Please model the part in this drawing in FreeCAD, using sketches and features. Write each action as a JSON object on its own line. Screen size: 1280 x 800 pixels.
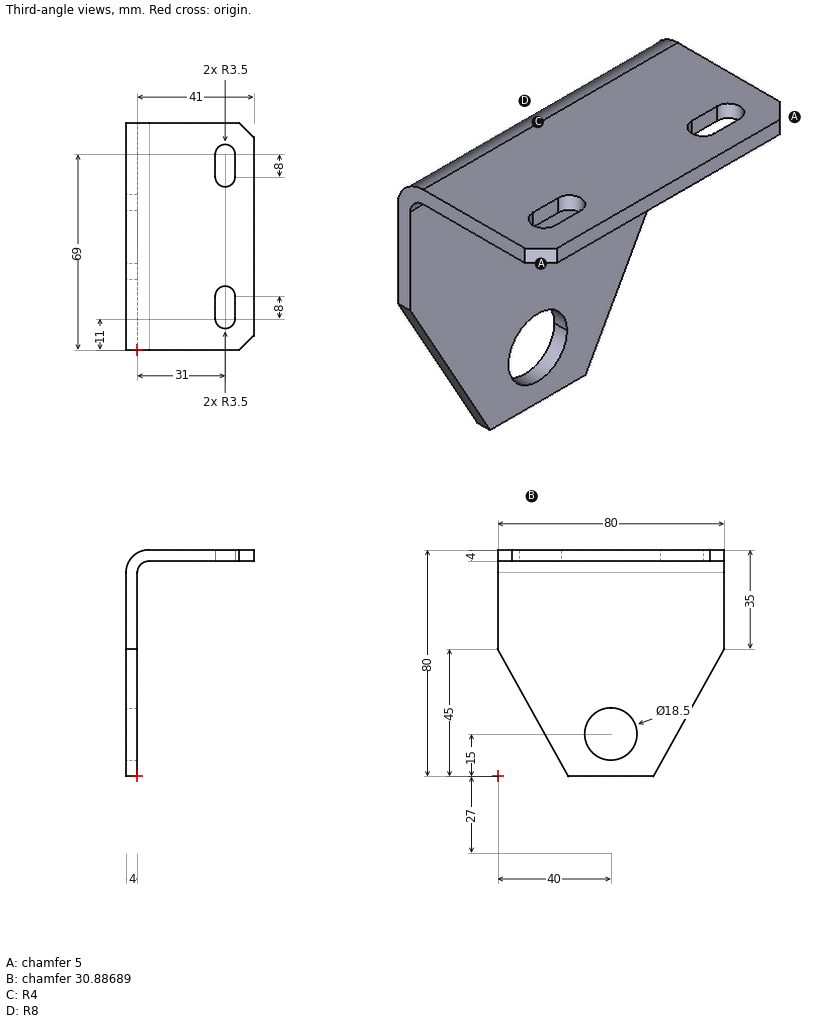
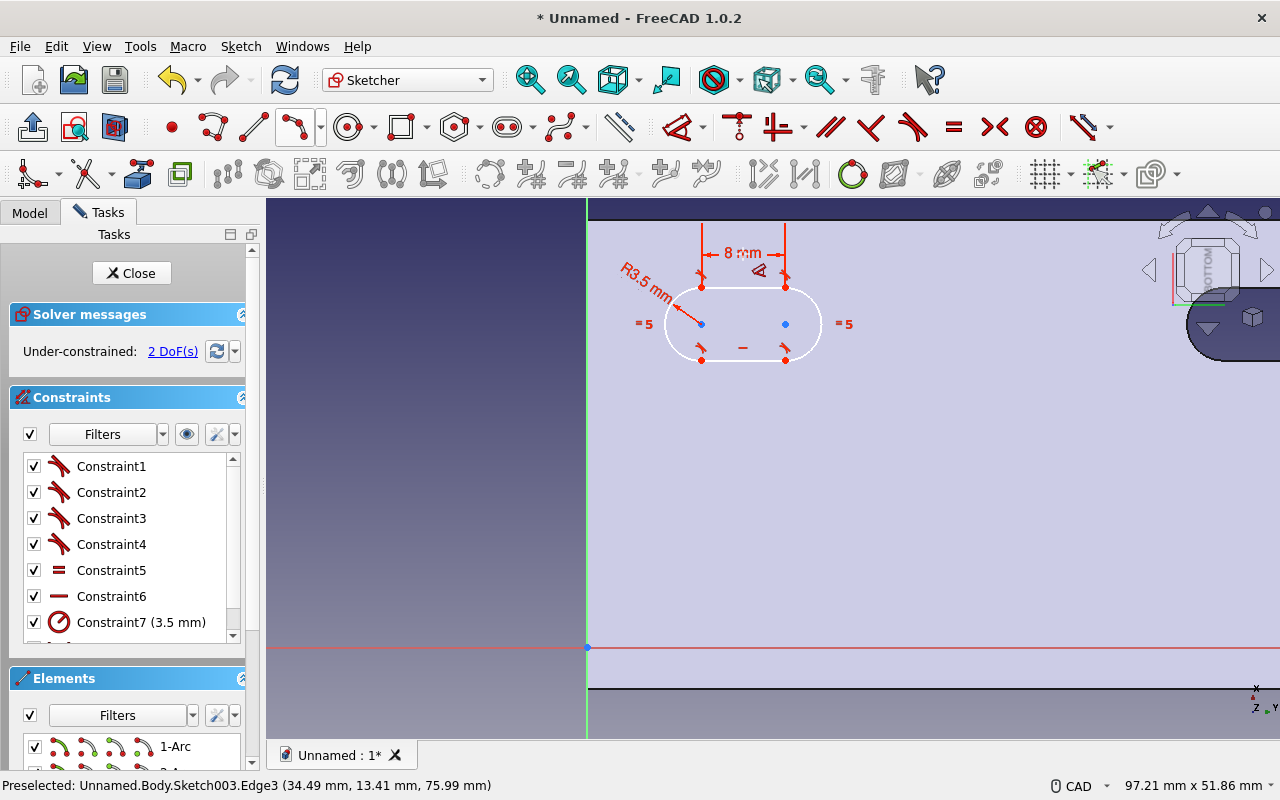
{"action": "left_click", "coordinate": [702, 288]}
{"action": "left_click", "coordinate": [644, 682]}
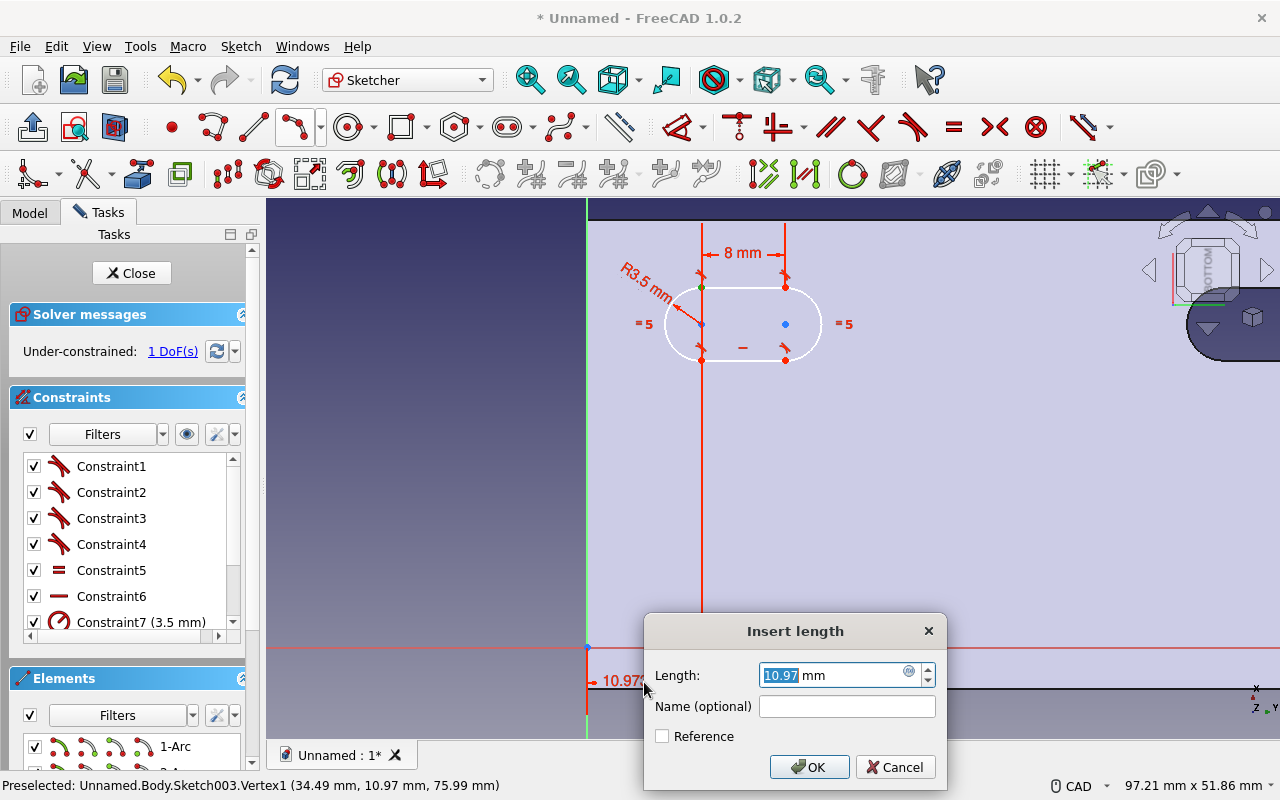
{"action": "type", "text": "11"}
{"action": "key", "text": "Return"}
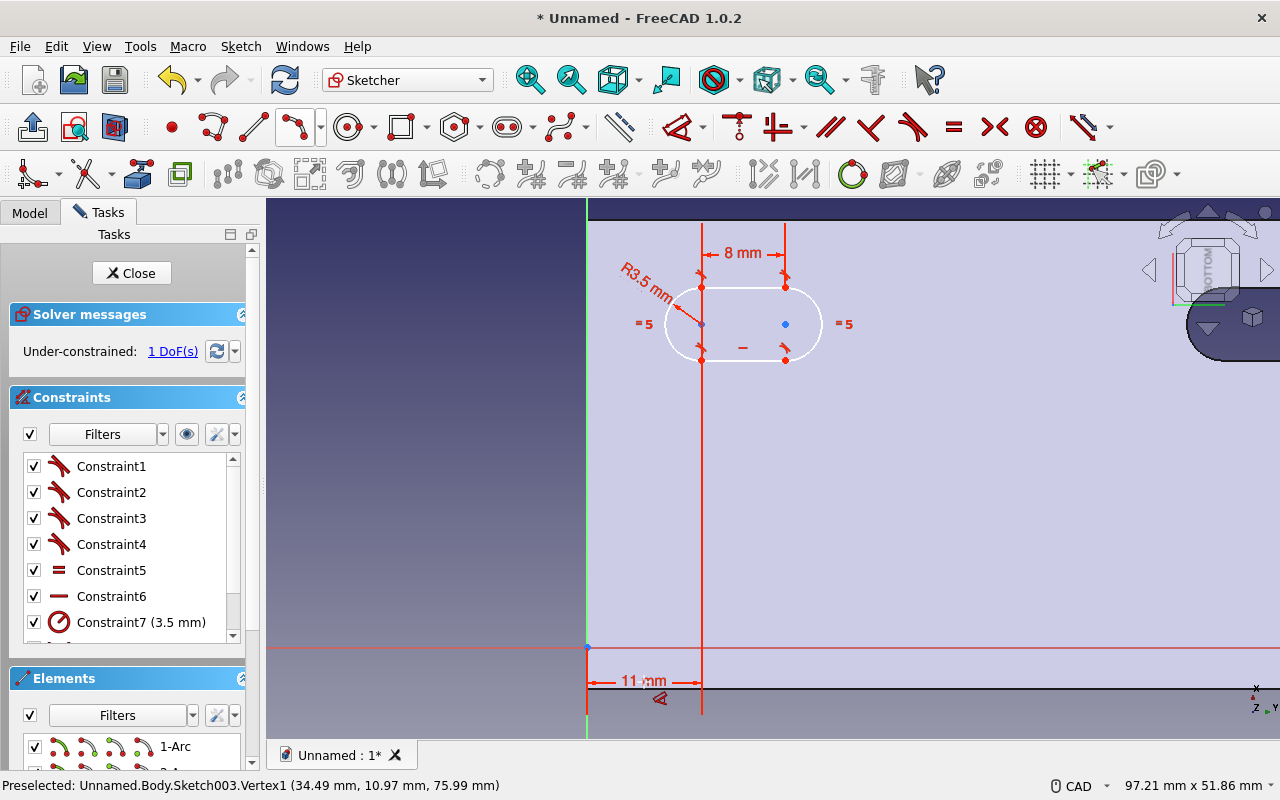
{"action": "left_click", "coordinate": [702, 324]}
{"action": "left_click", "coordinate": [553, 486]}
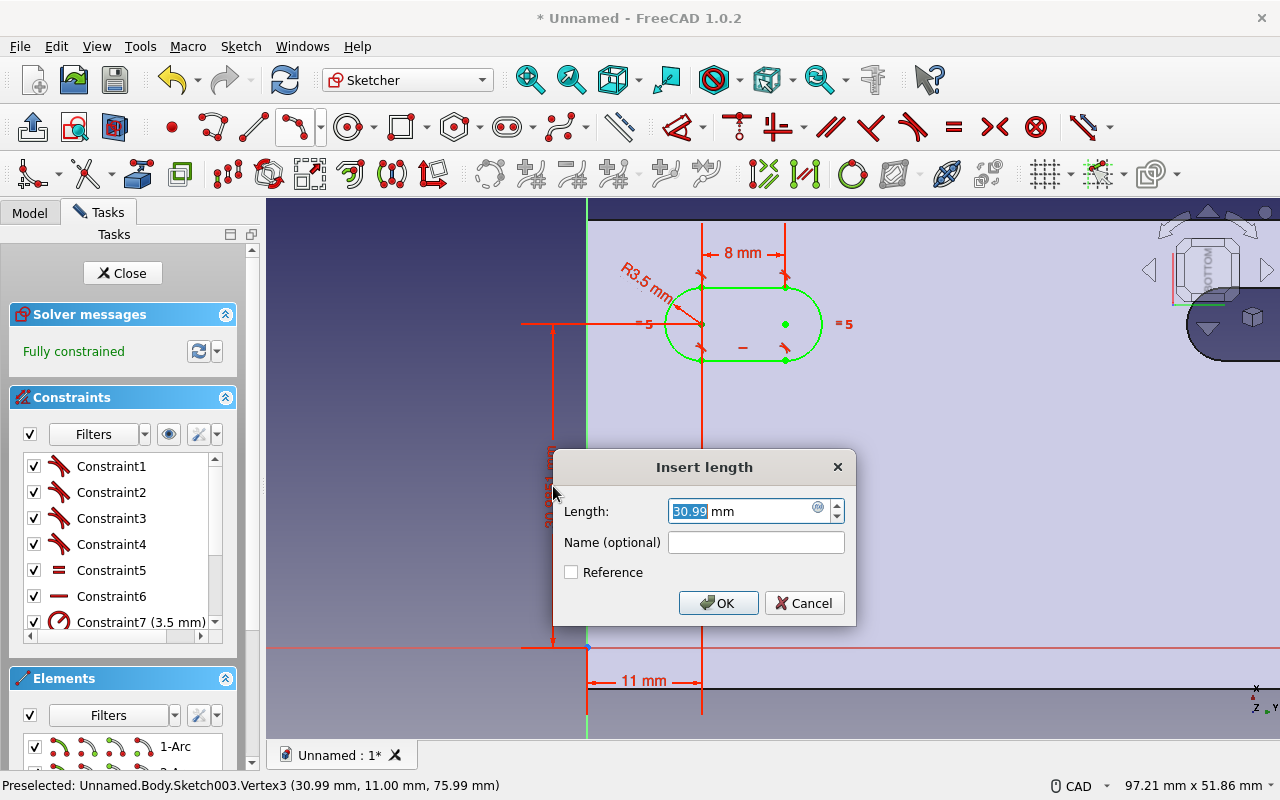
{"action": "type", "text": "31"}
{"action": "key", "text": "Return"}
{"action": "key", "text": "Escape"}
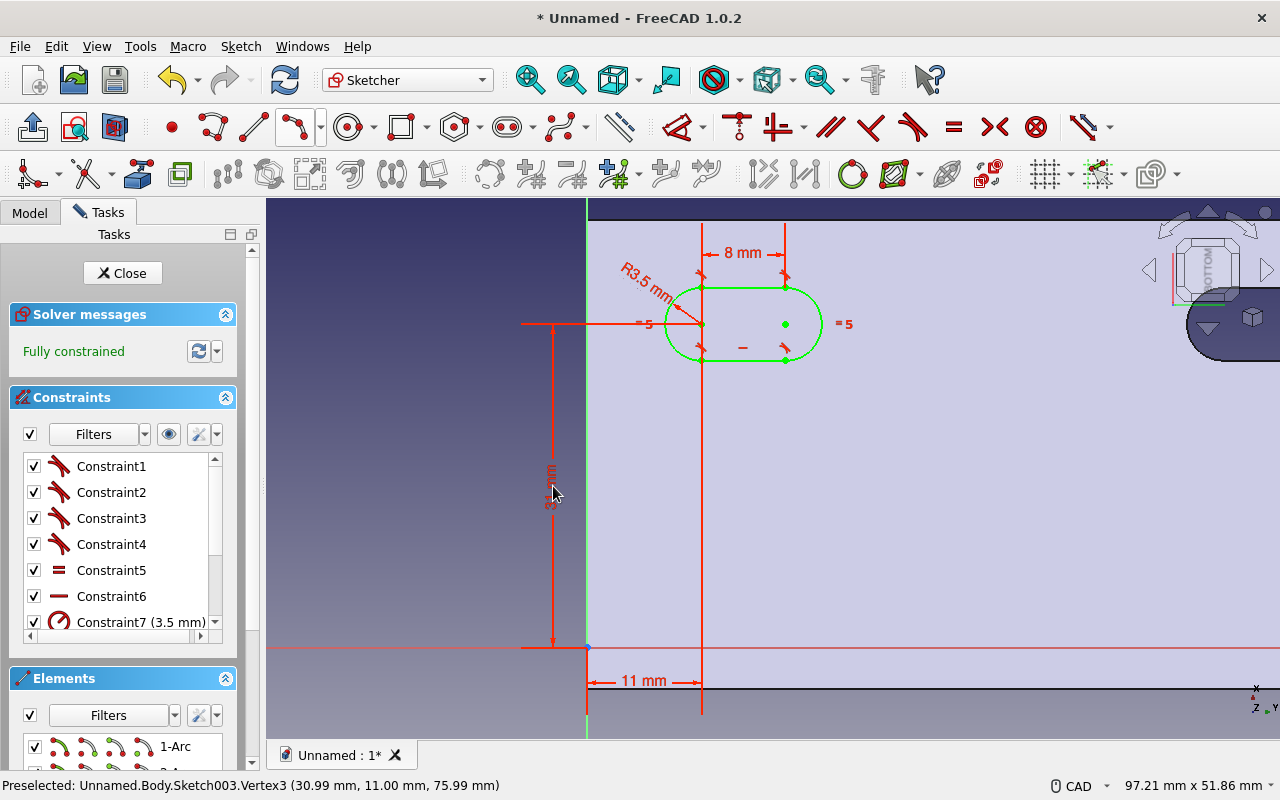
{"action": "left_click", "coordinate": [123, 273]}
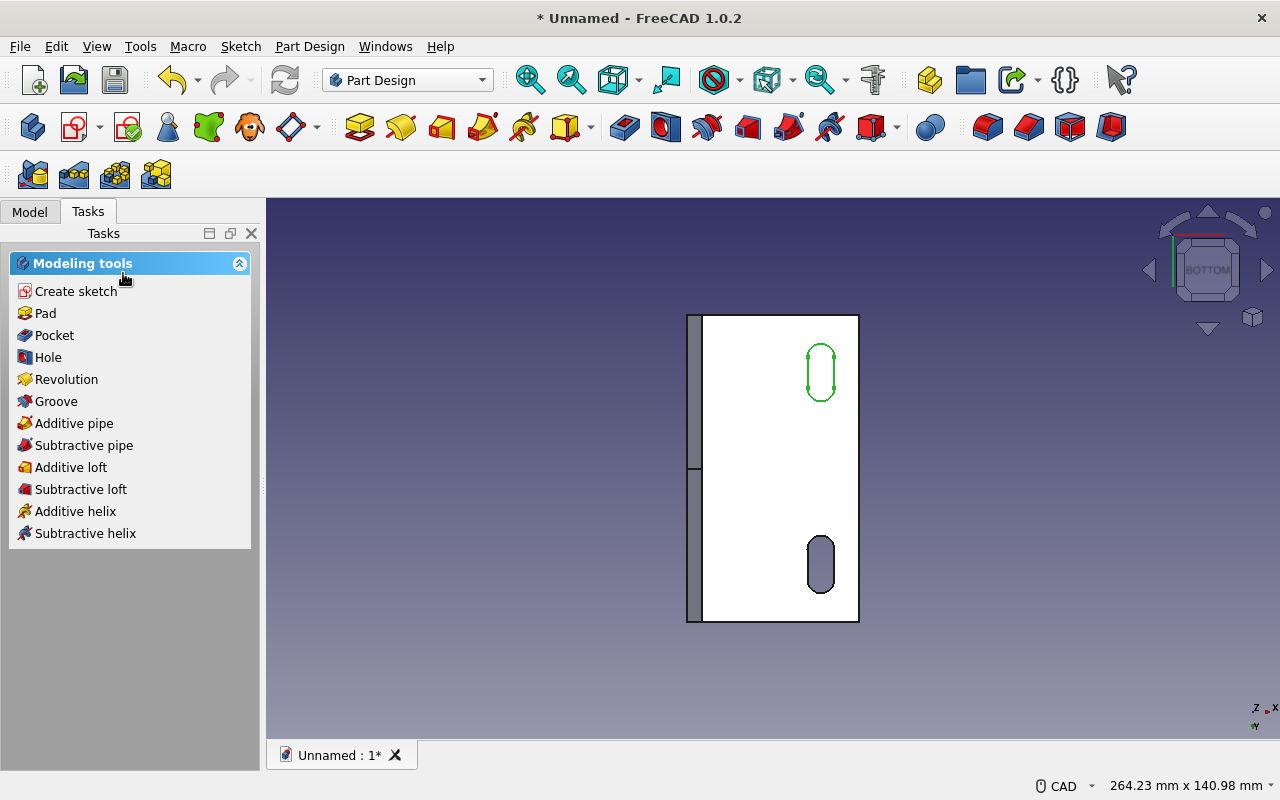
{"action": "left_click", "coordinate": [625, 128]}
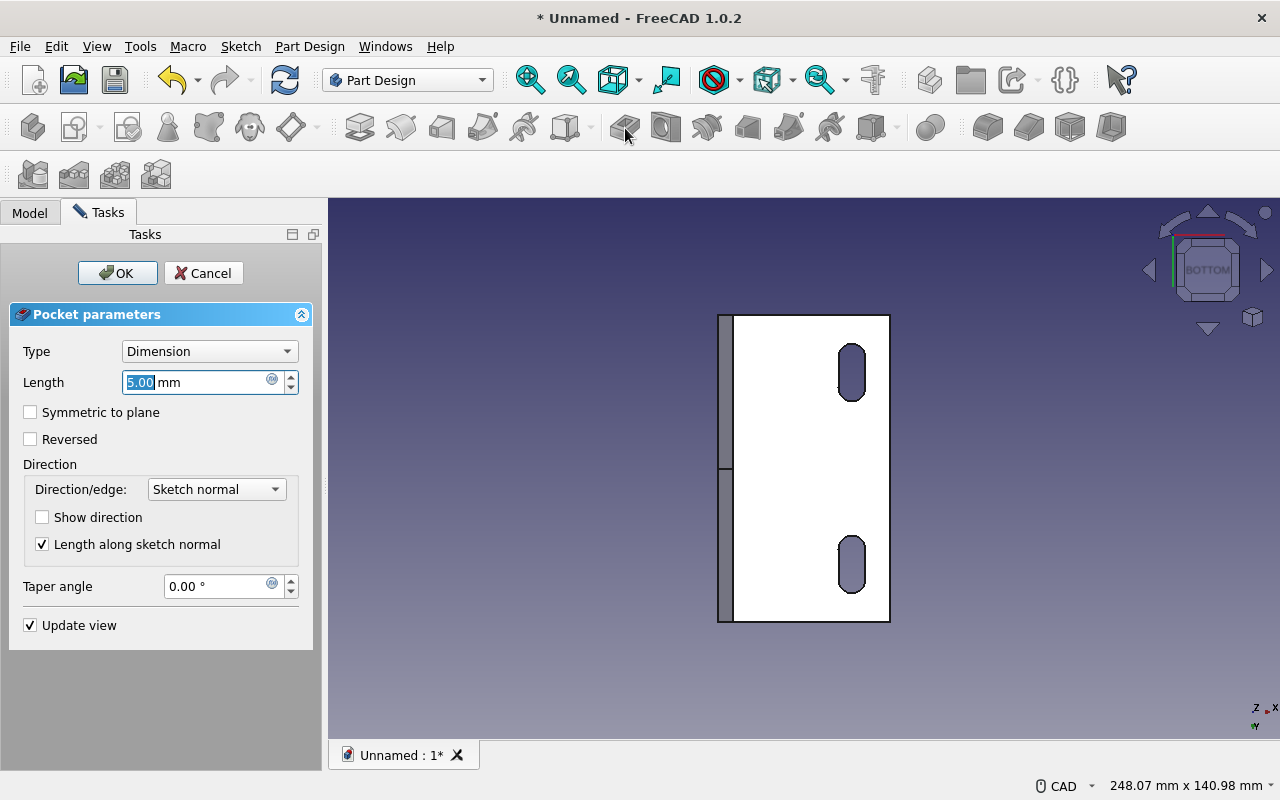
{"action": "left_click", "coordinate": [210, 352]}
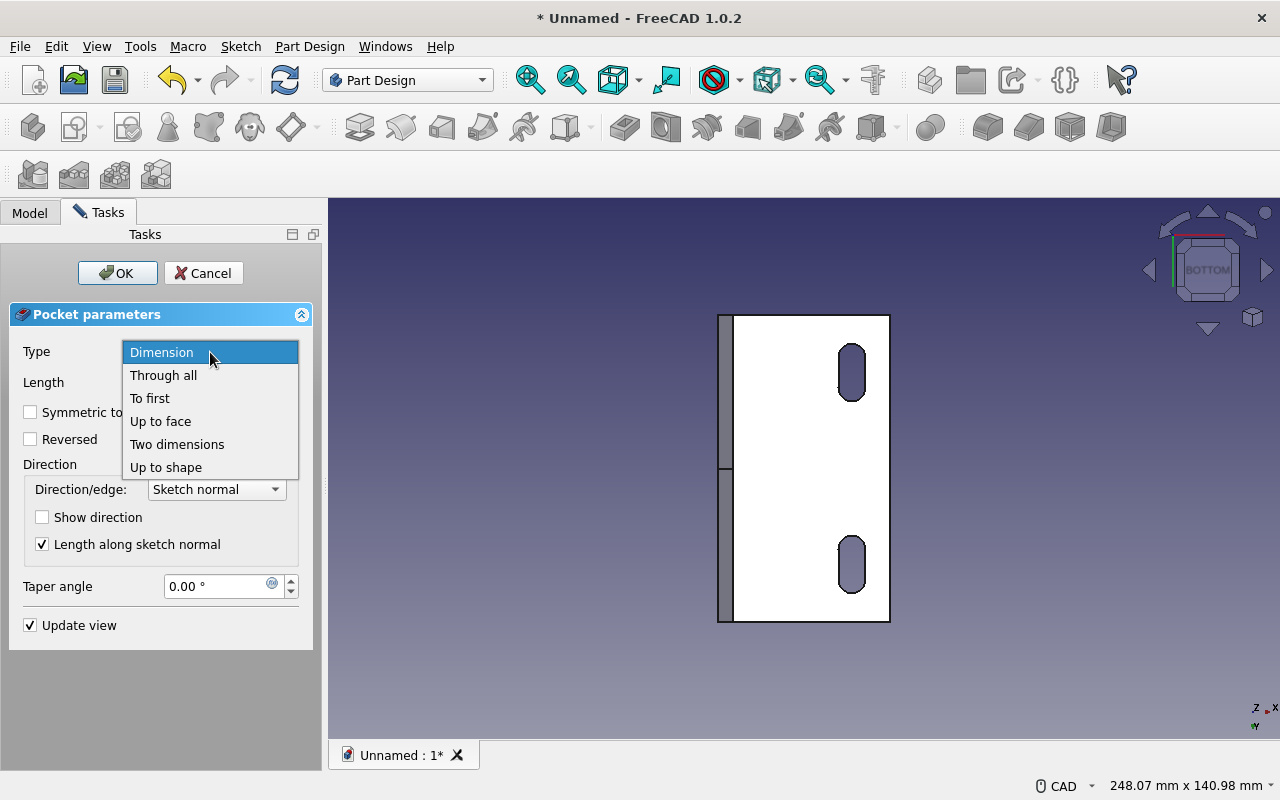
{"action": "left_click", "coordinate": [208, 376]}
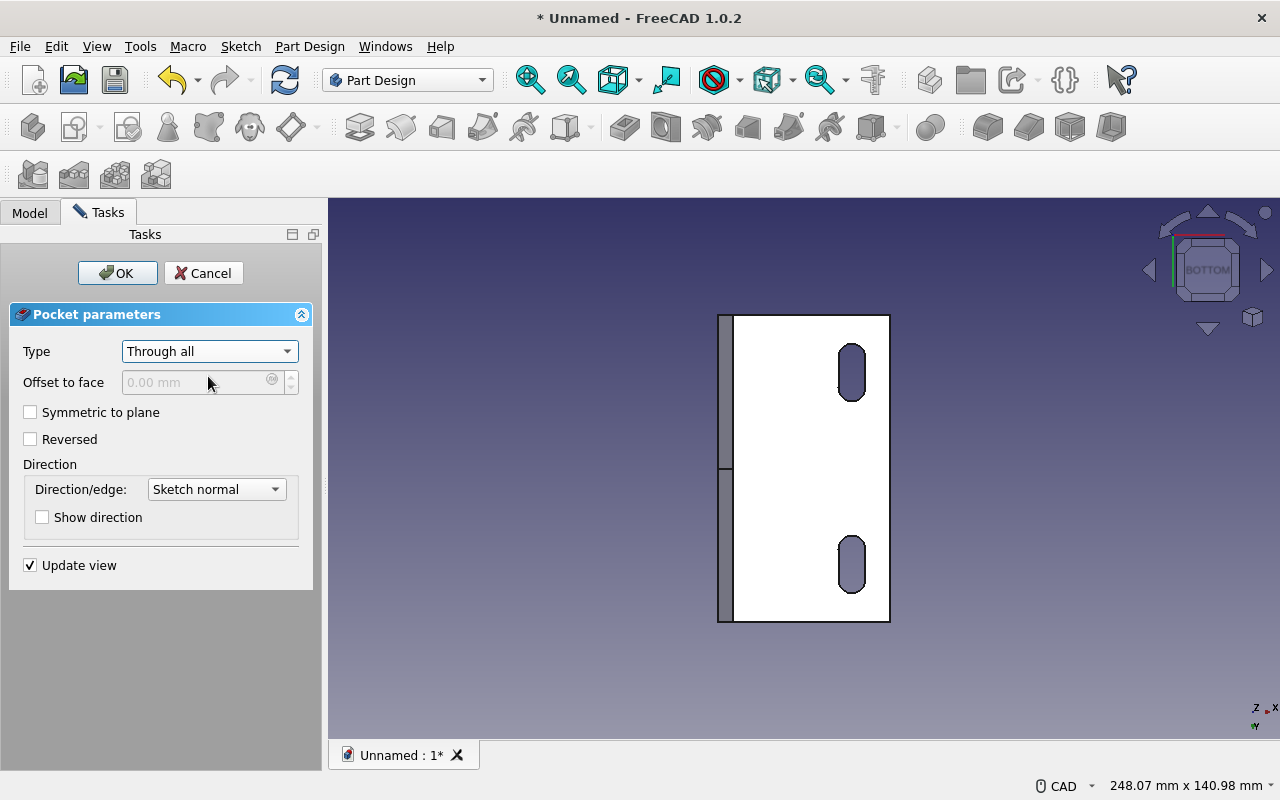
{"action": "left_click", "coordinate": [118, 273]}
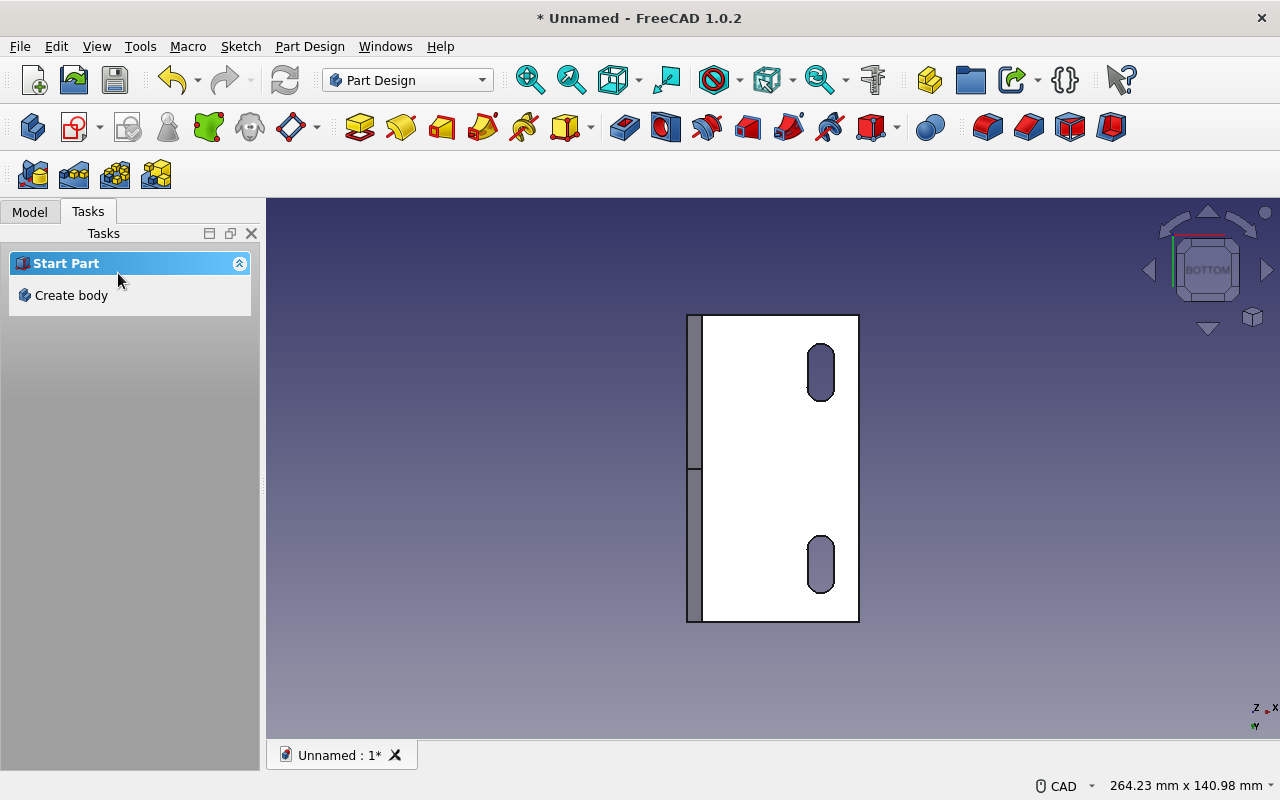
{"action": "key", "text": "0"}